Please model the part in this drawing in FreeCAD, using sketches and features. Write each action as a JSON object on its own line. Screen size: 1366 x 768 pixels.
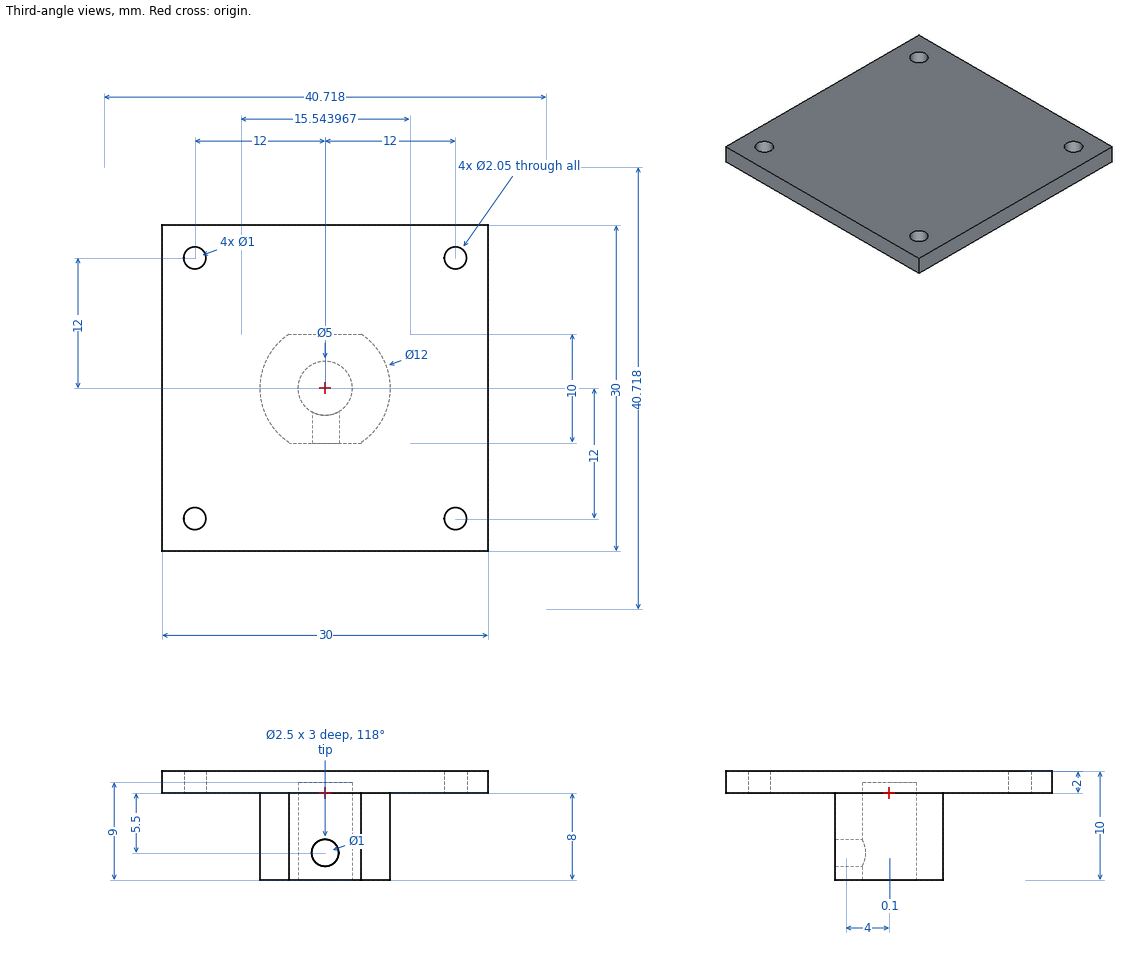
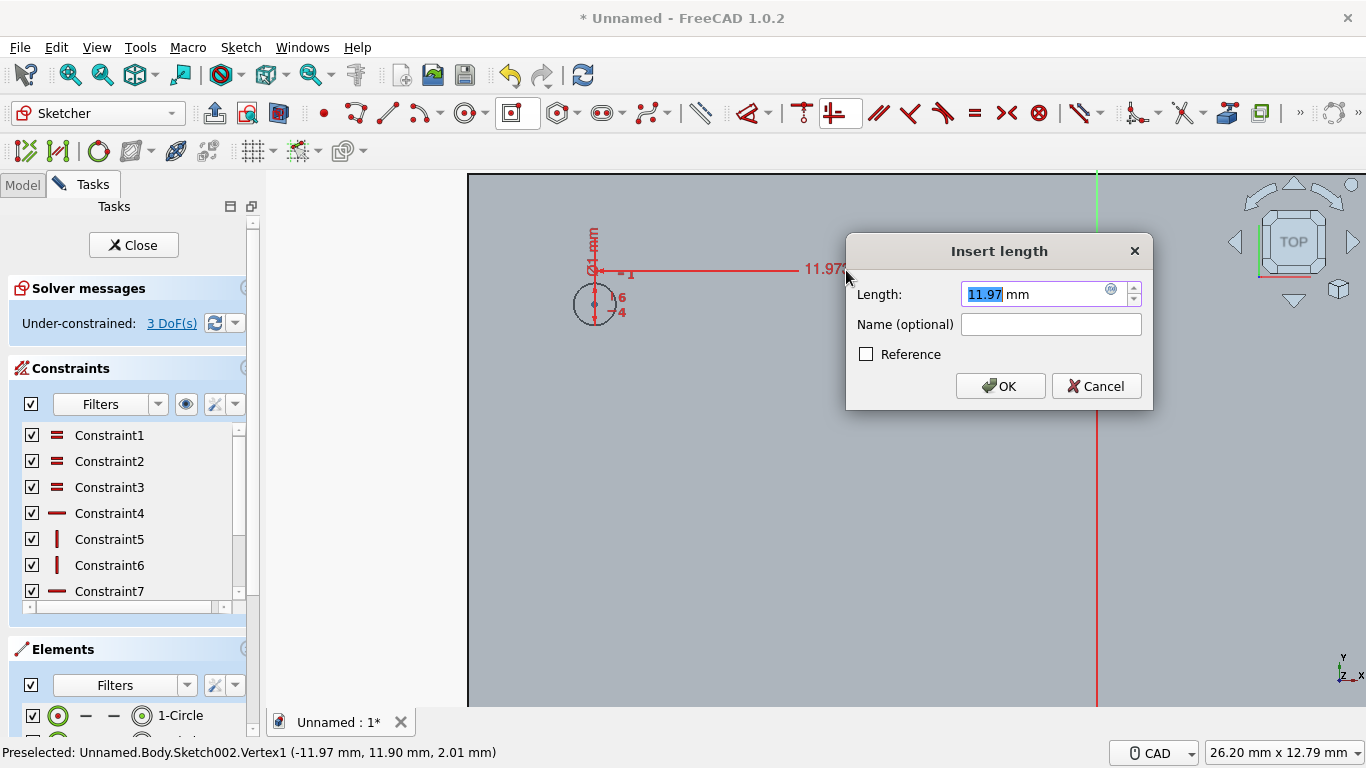
{"action": "type", "text": "12"}
{"action": "key", "text": "Return"}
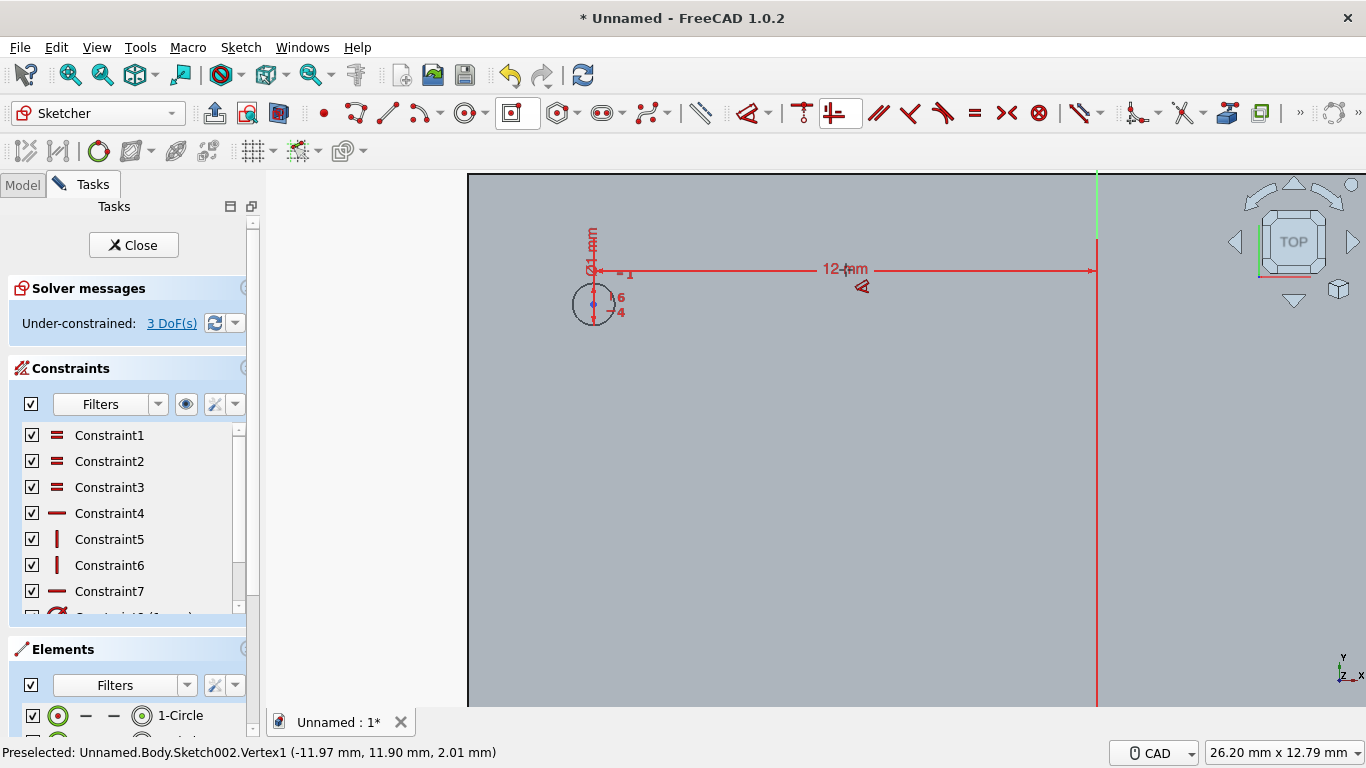
{"action": "left_click", "coordinate": [594, 304]}
{"action": "left_click", "coordinate": [560, 492]}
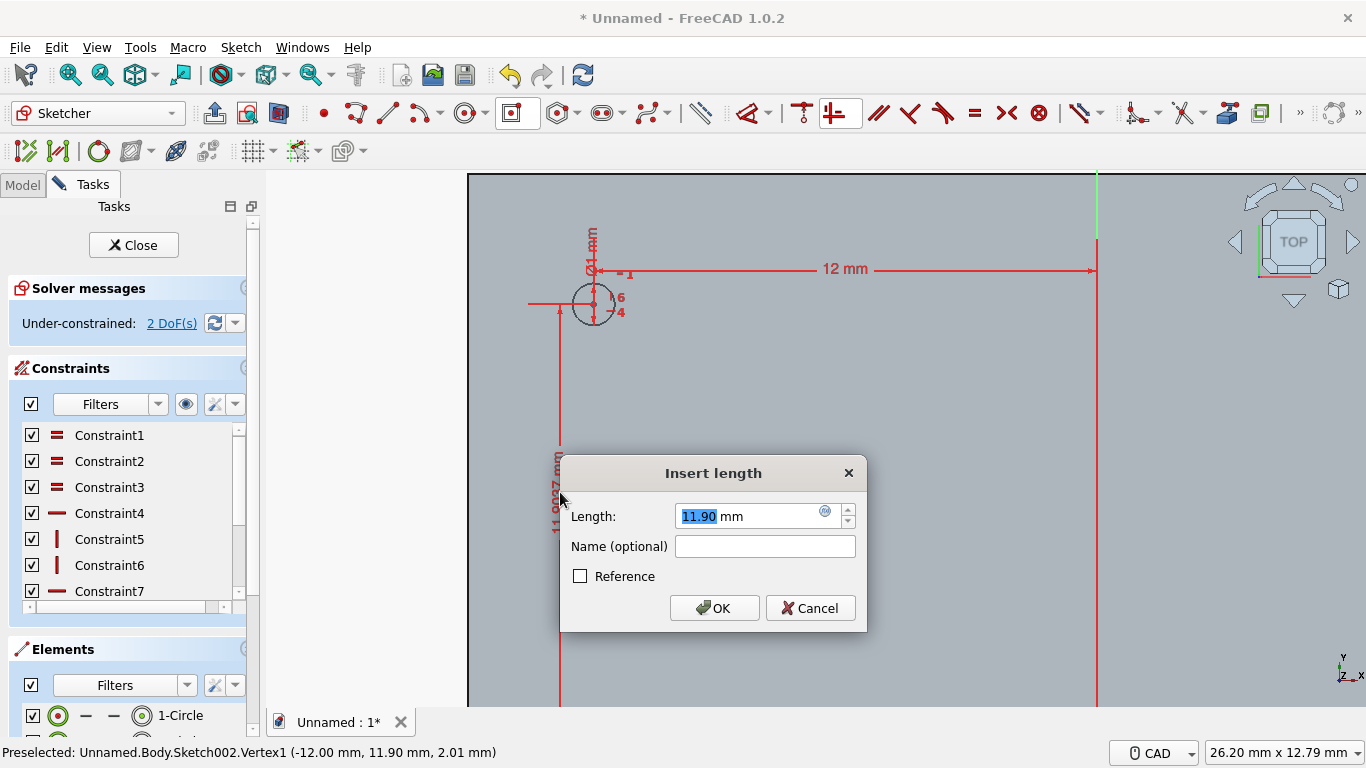
{"action": "type", "text": "12"}
{"action": "key", "text": "Return"}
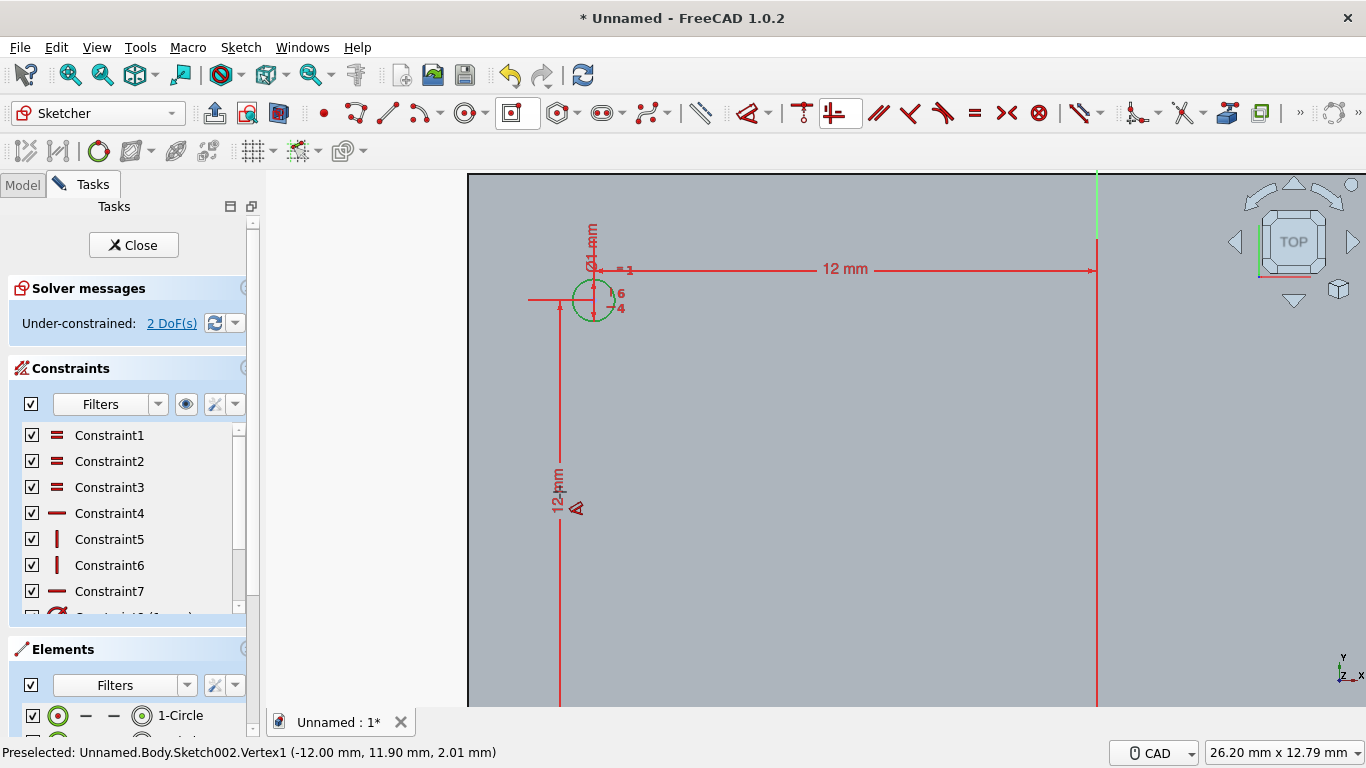
{"action": "scroll", "coordinate": [597, 281], "scroll_direction": "down", "scroll_amount": 6}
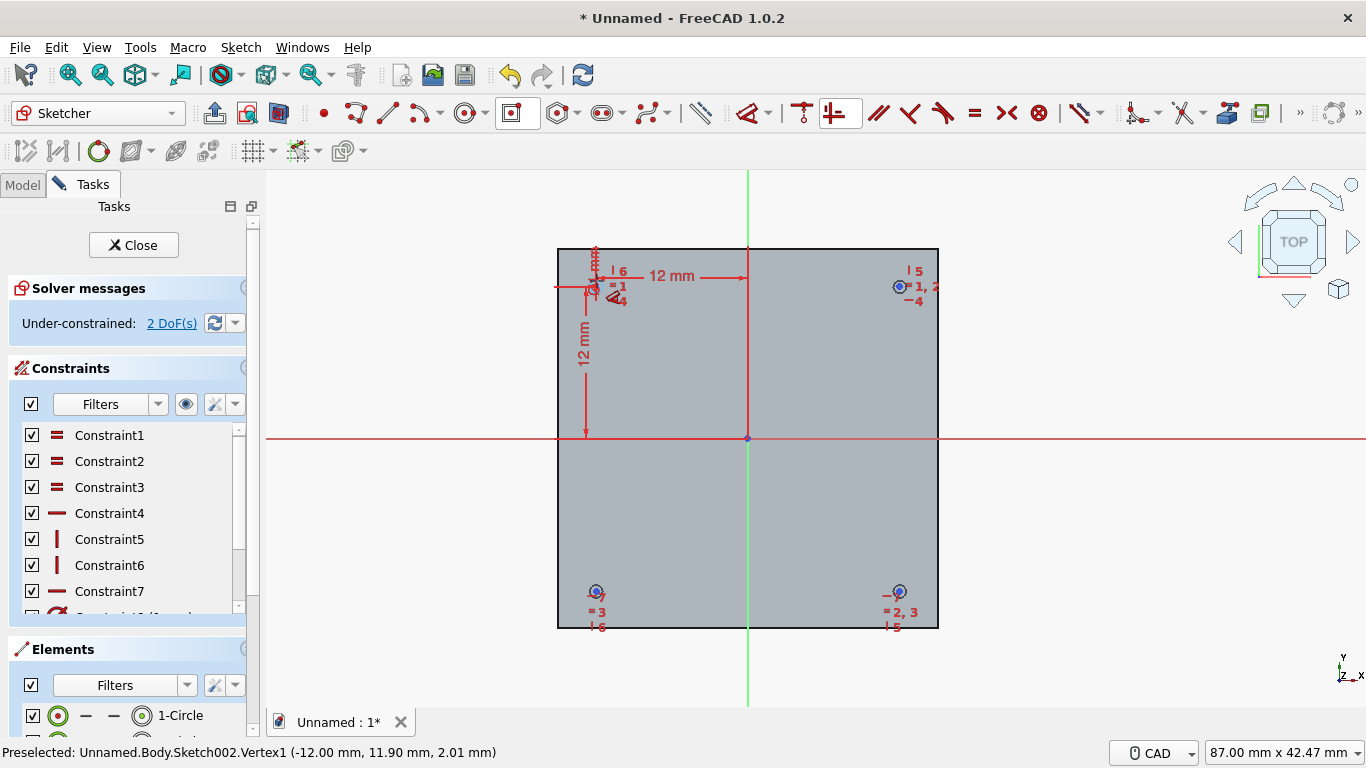
{"action": "left_click", "coordinate": [900, 287]}
{"action": "left_click", "coordinate": [824, 253]}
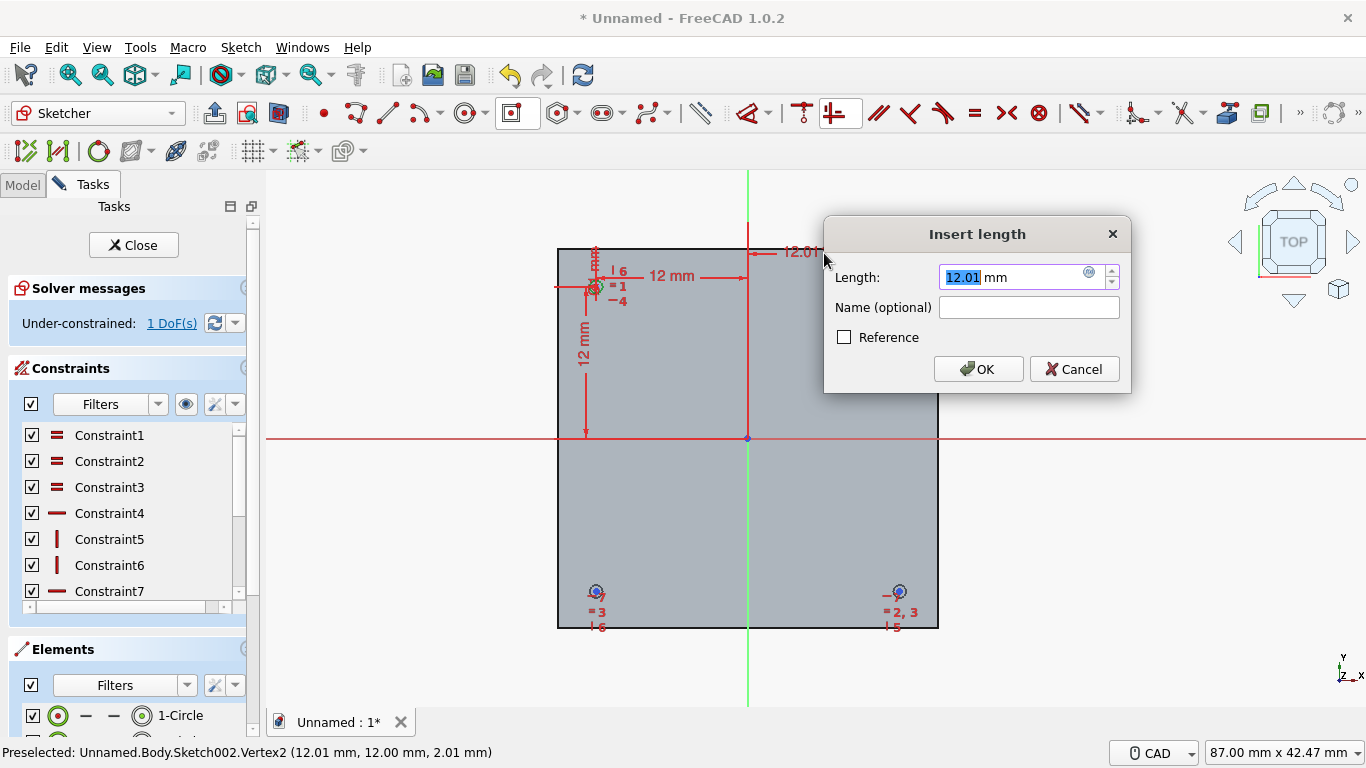
{"action": "type", "text": "12"}
{"action": "key", "text": "Return"}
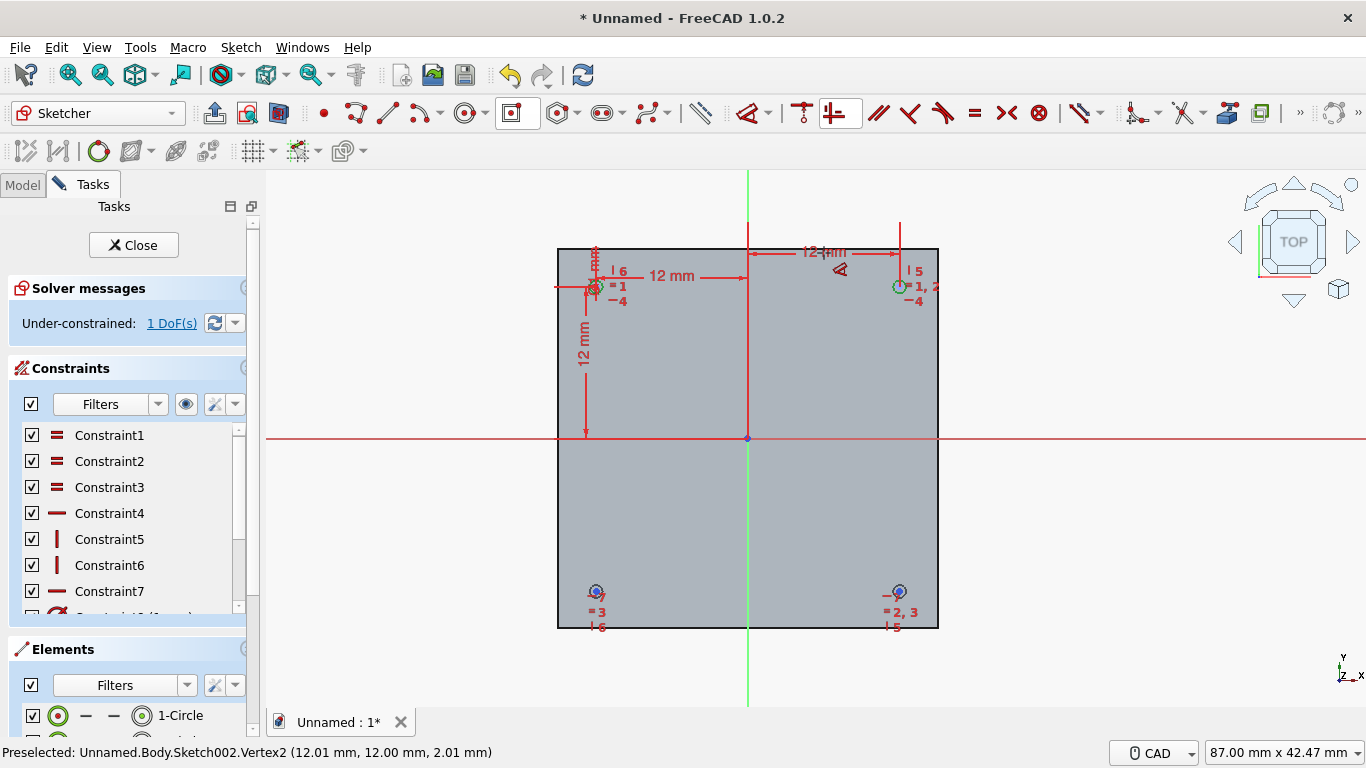
{"action": "left_click", "coordinate": [900, 591]}
{"action": "left_click", "coordinate": [934, 515]}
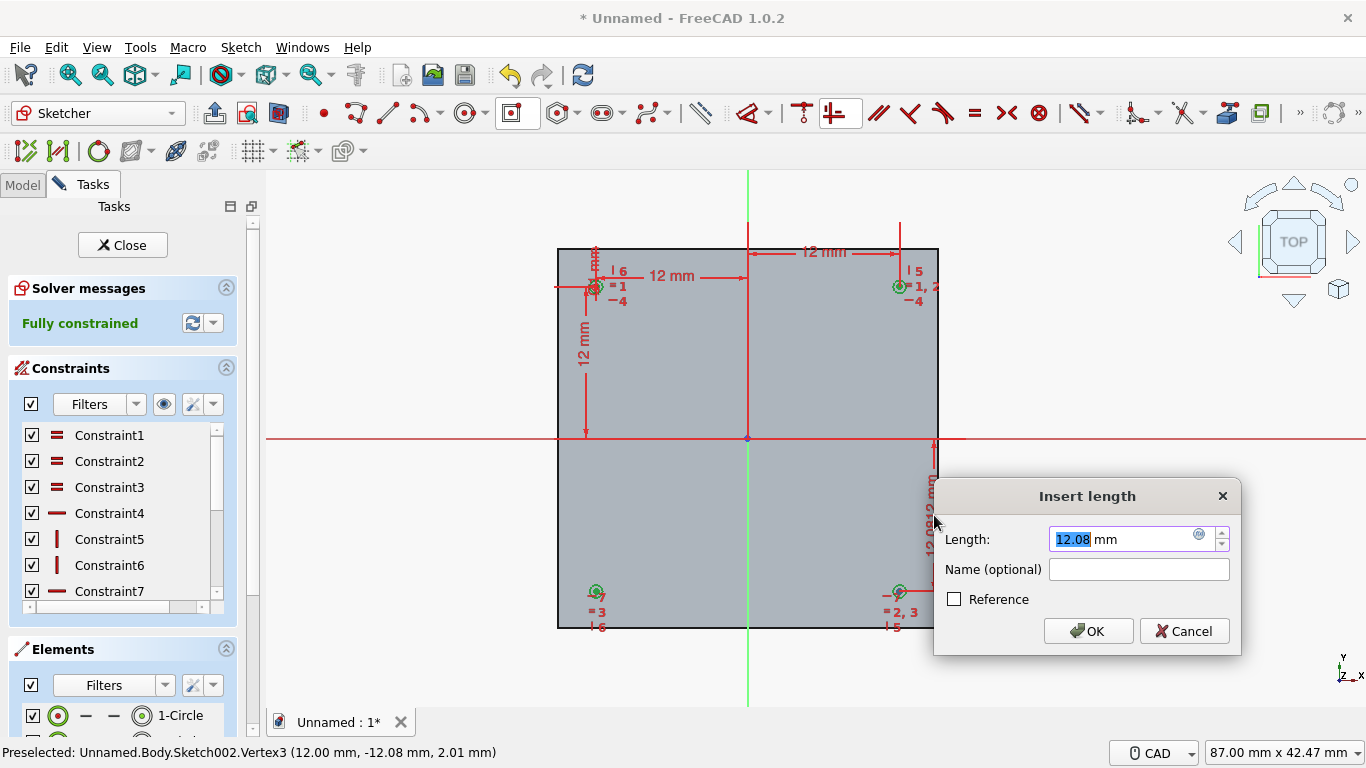
{"action": "type", "text": "12"}
{"action": "key", "text": "Return"}
{"action": "key", "text": "Escape"}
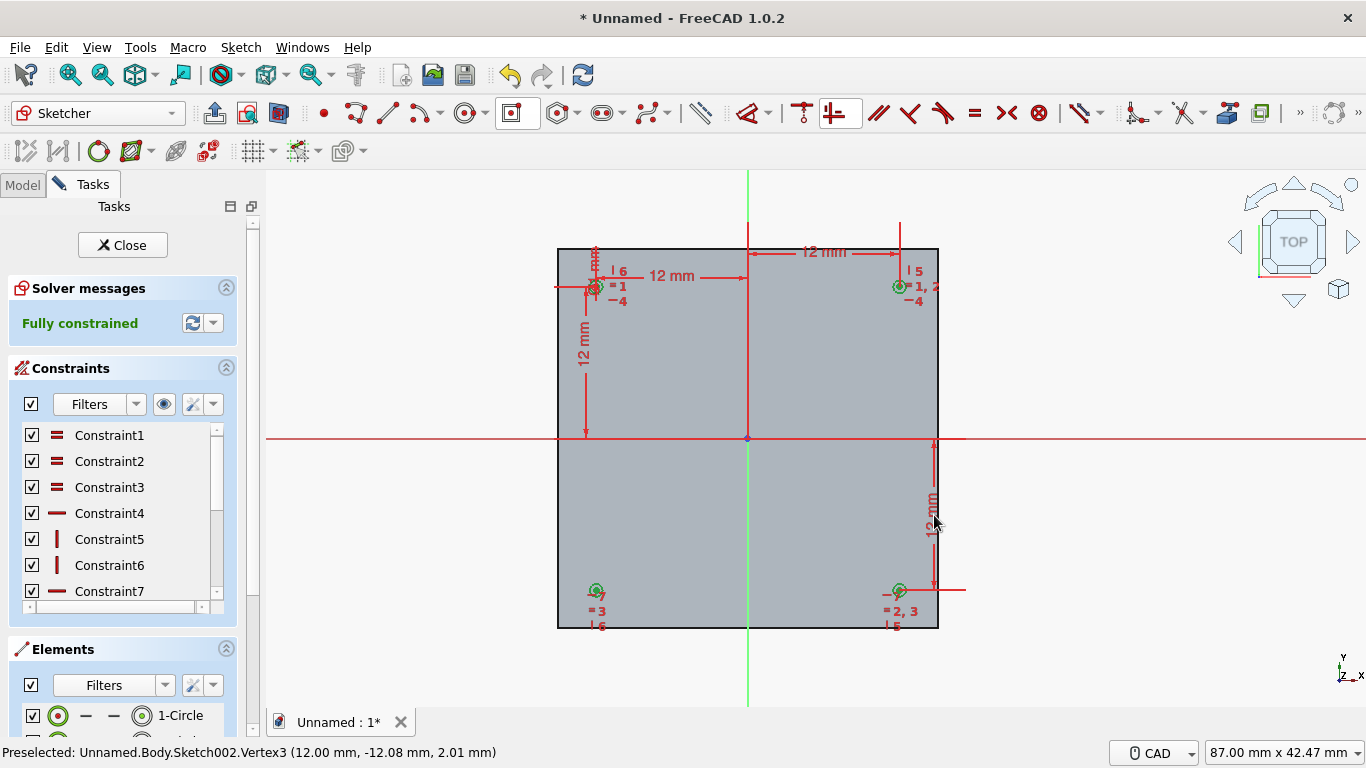
{"action": "left_click", "coordinate": [123, 245]}